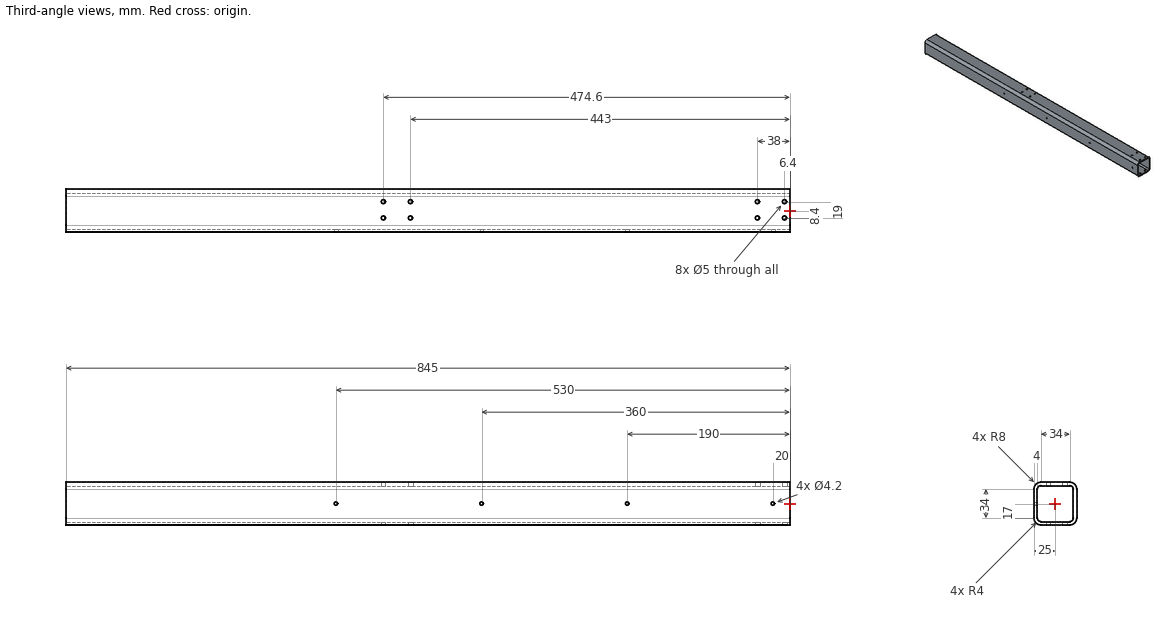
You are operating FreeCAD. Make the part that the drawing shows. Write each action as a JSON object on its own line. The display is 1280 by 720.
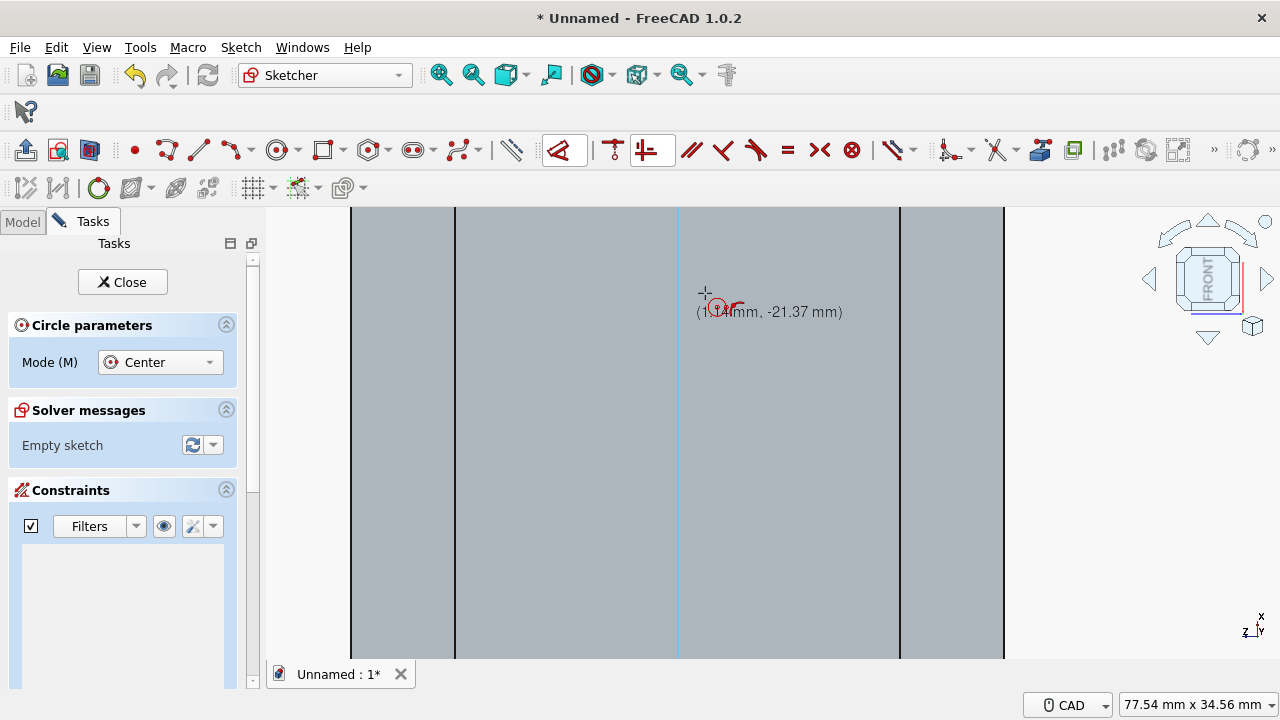
{"action": "scroll", "coordinate": [706, 302], "scroll_direction": "down", "scroll_amount": 16}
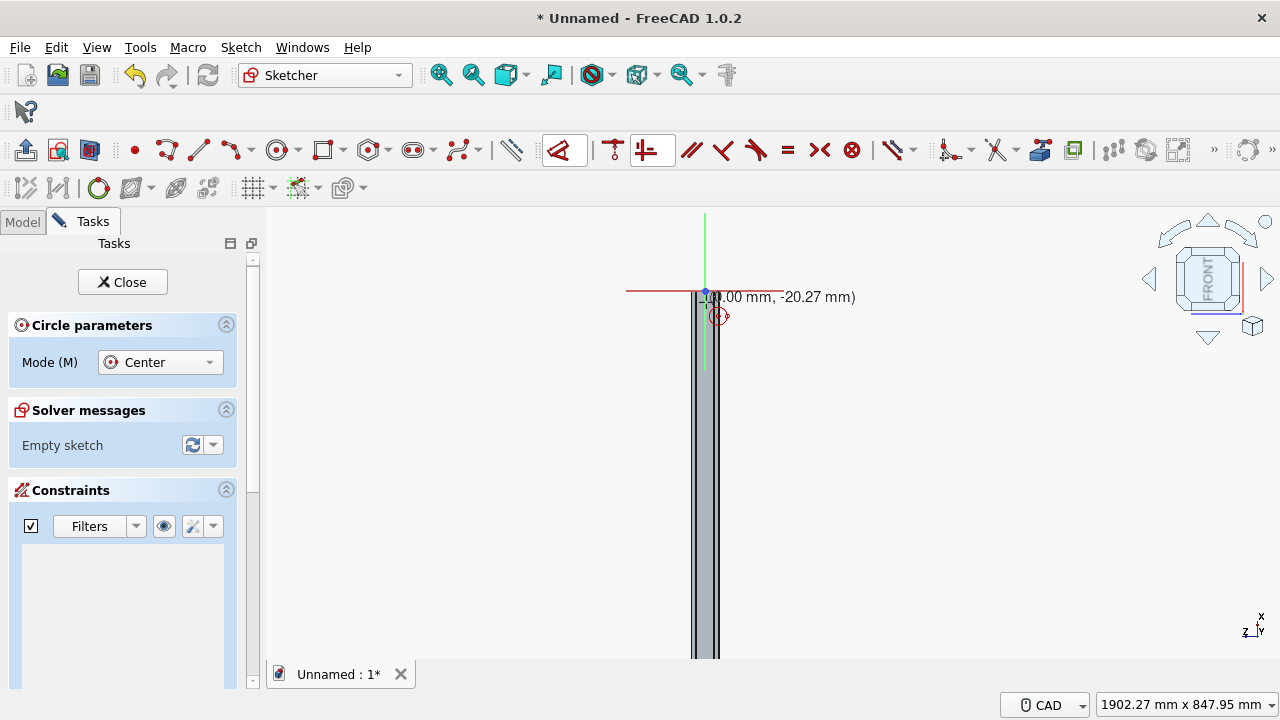
{"action": "scroll", "coordinate": [705, 302], "scroll_direction": "up", "scroll_amount": 2}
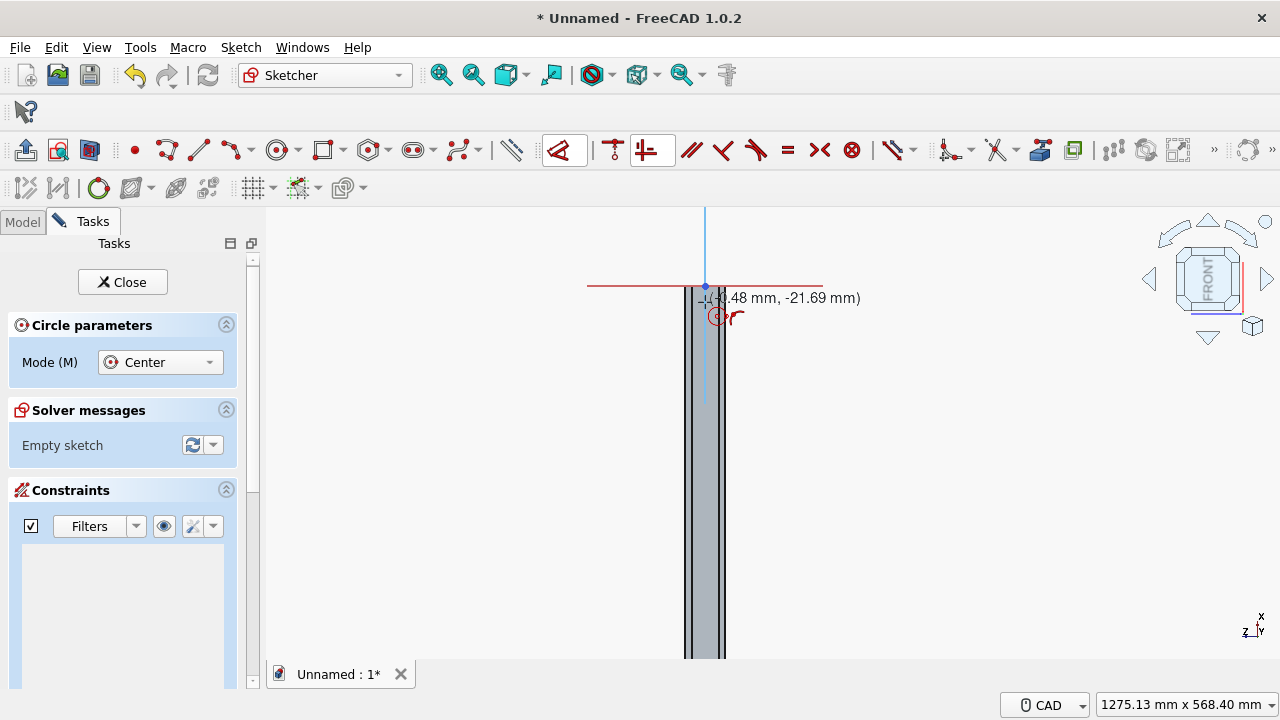
{"action": "left_click", "coordinate": [705, 302]}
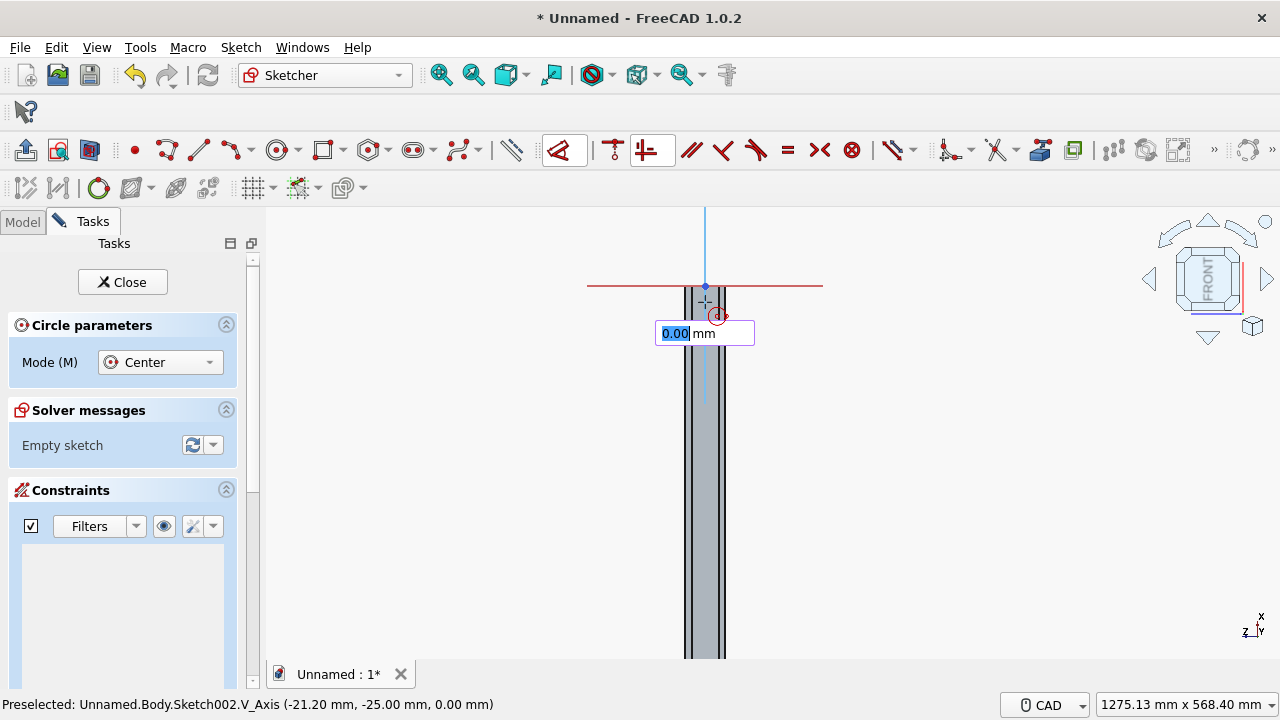
{"action": "scroll", "coordinate": [707, 301], "scroll_direction": "up", "scroll_amount": 12}
{"action": "mouse_move", "coordinate": [700, 304]}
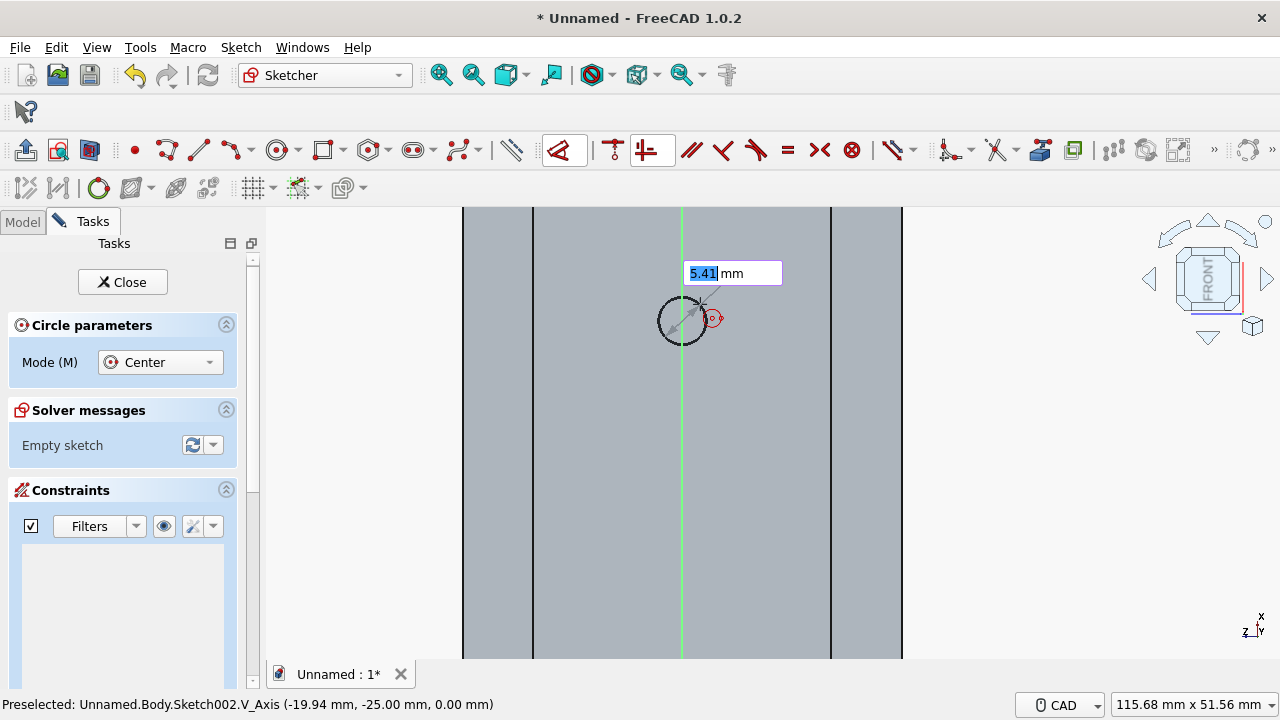
{"action": "type", "text": "4.2"}
{"action": "key", "text": "Return"}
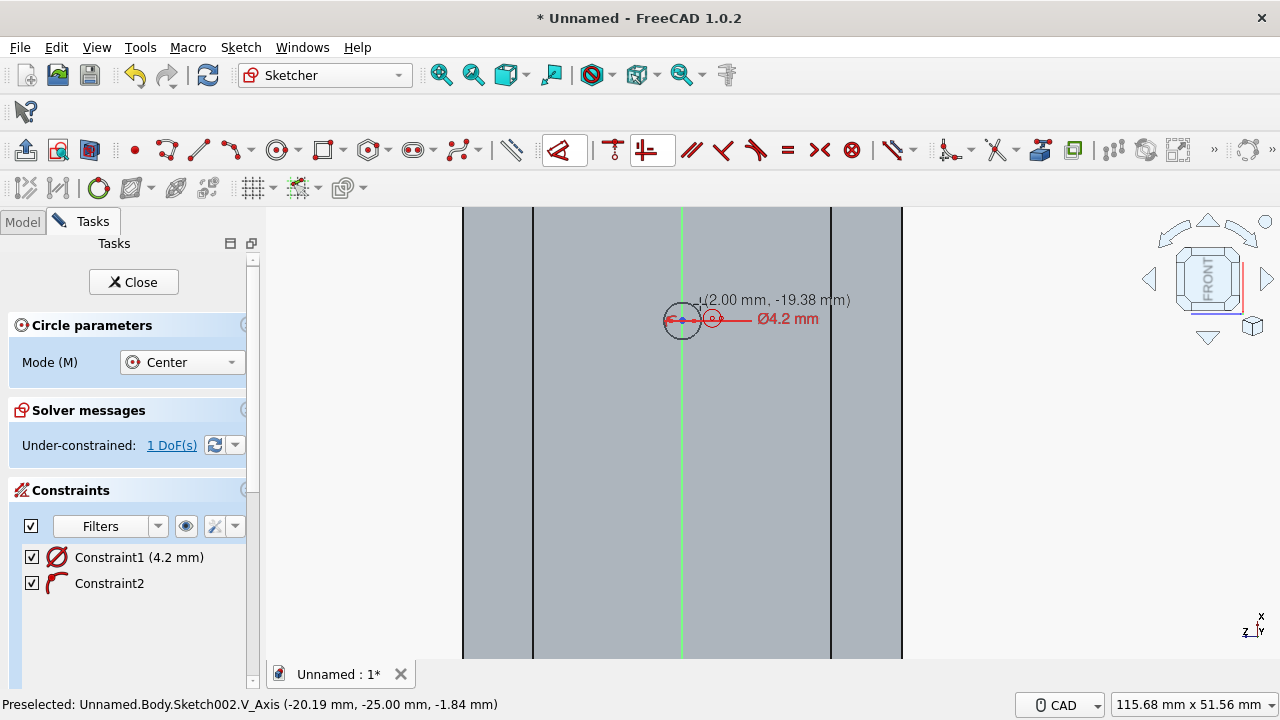
{"action": "scroll", "coordinate": [706, 301], "scroll_direction": "down", "scroll_amount": 14}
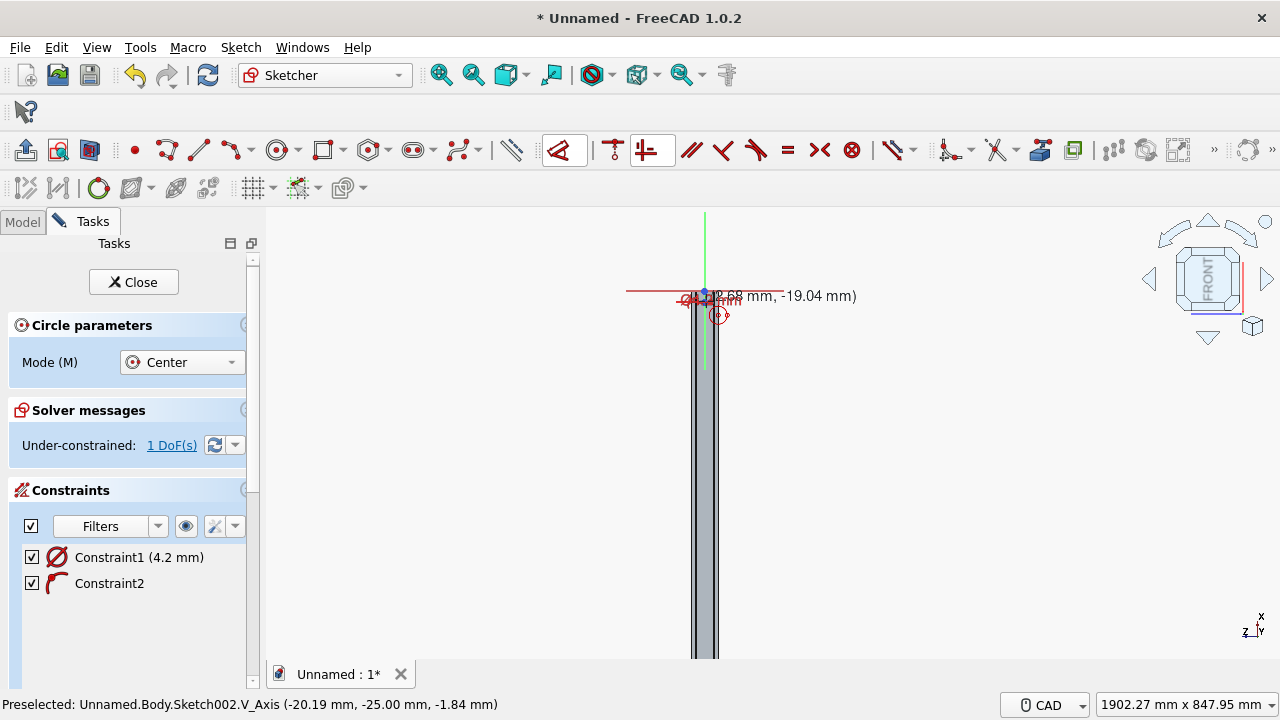
{"action": "scroll", "coordinate": [705, 392], "scroll_direction": "up", "scroll_amount": 16}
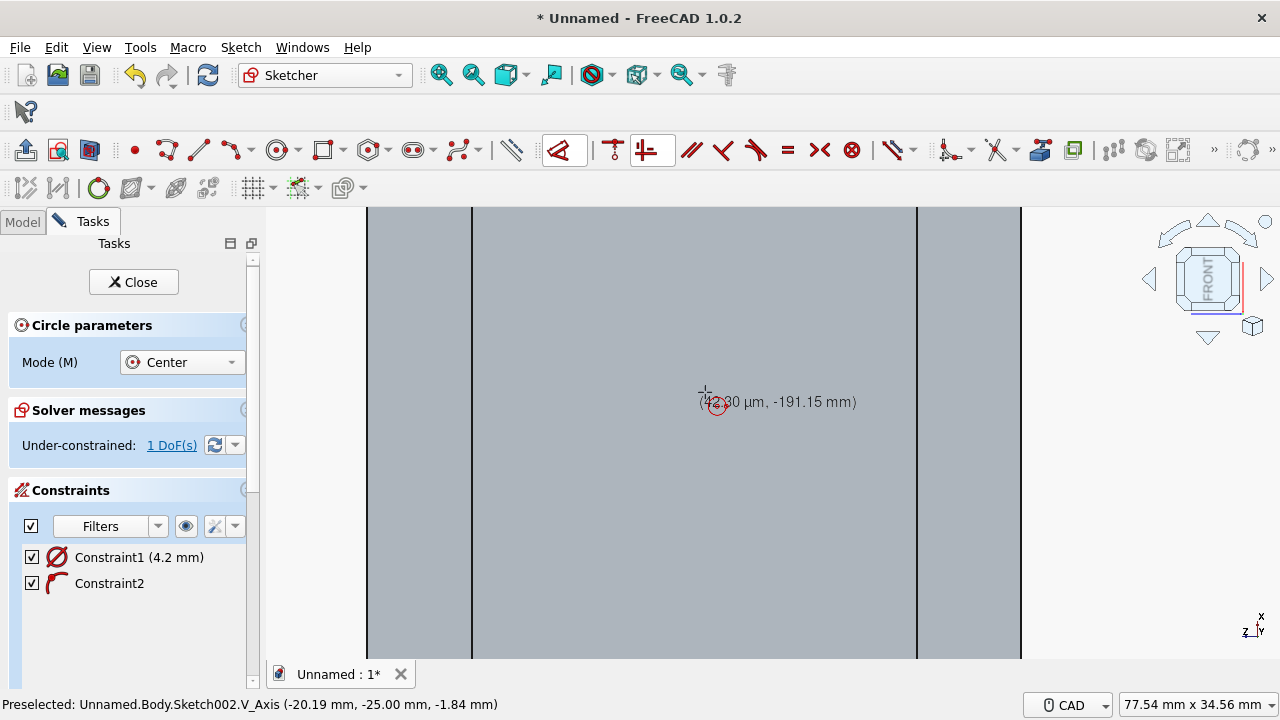
{"action": "scroll", "coordinate": [705, 392], "scroll_direction": "down", "scroll_amount": 16}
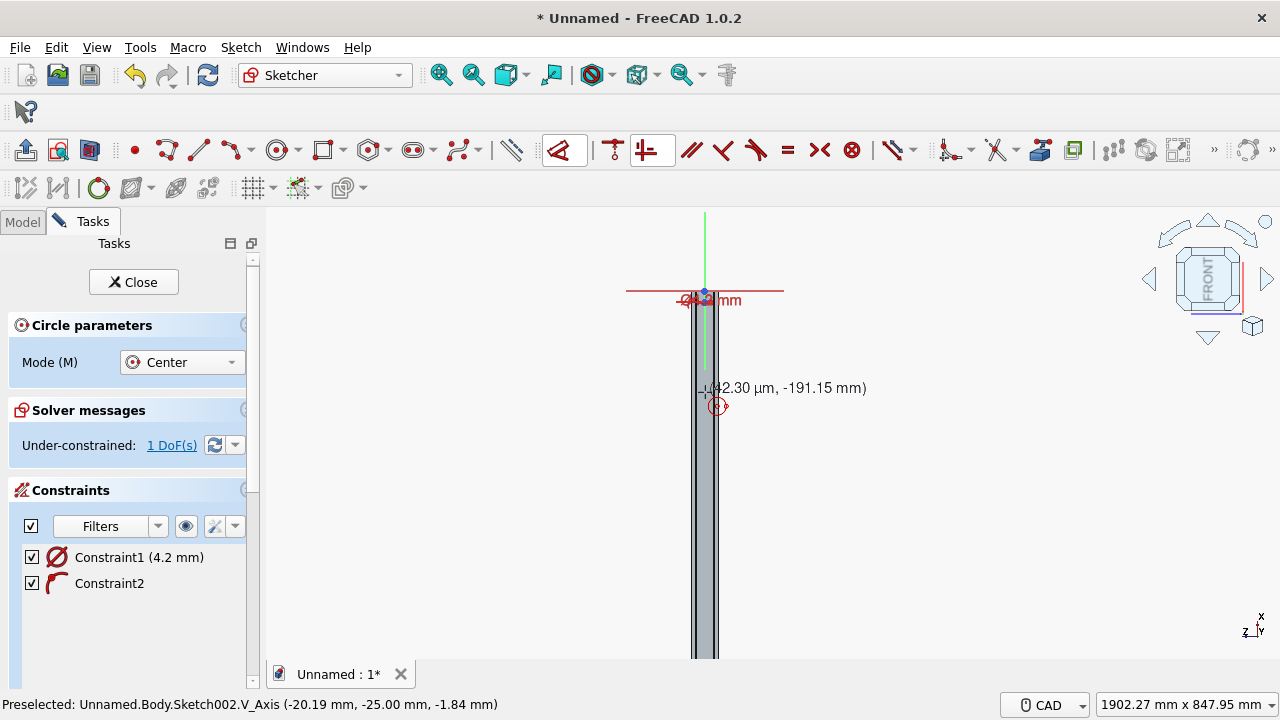
{"action": "left_click", "coordinate": [705, 392]}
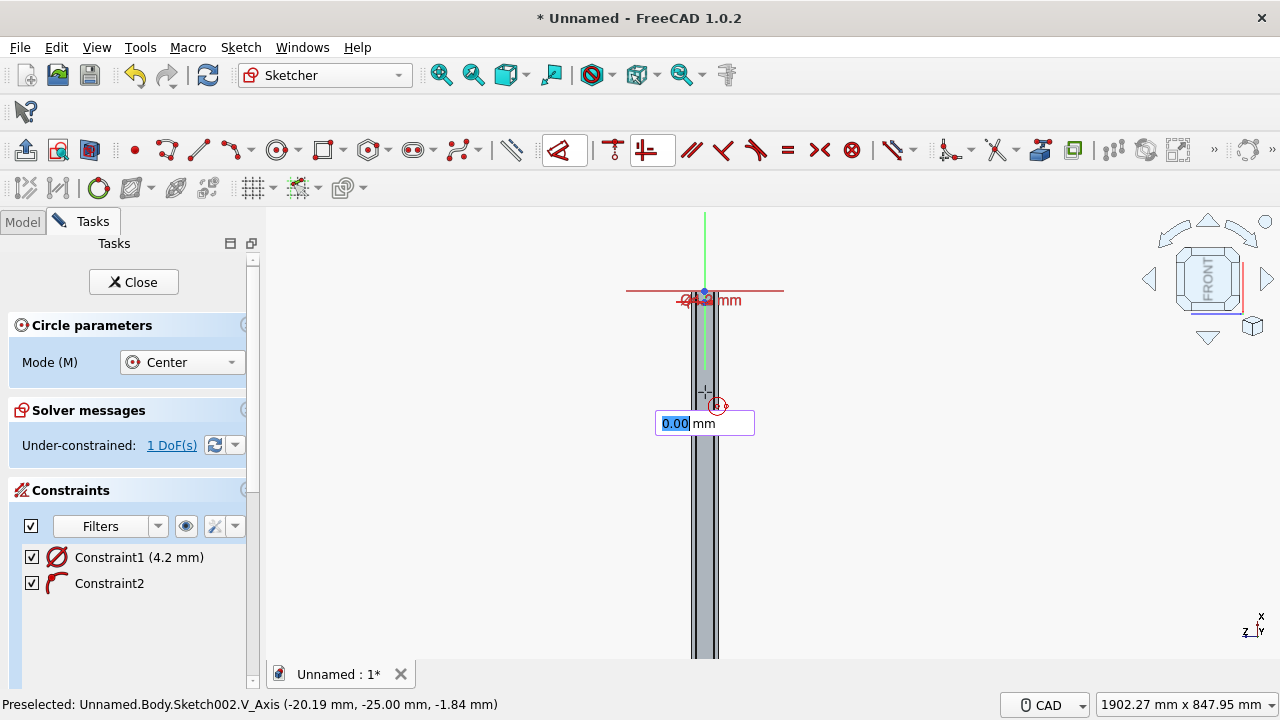
{"action": "scroll", "coordinate": [706, 392], "scroll_direction": "up", "scroll_amount": 14}
{"action": "mouse_move", "coordinate": [700, 386]}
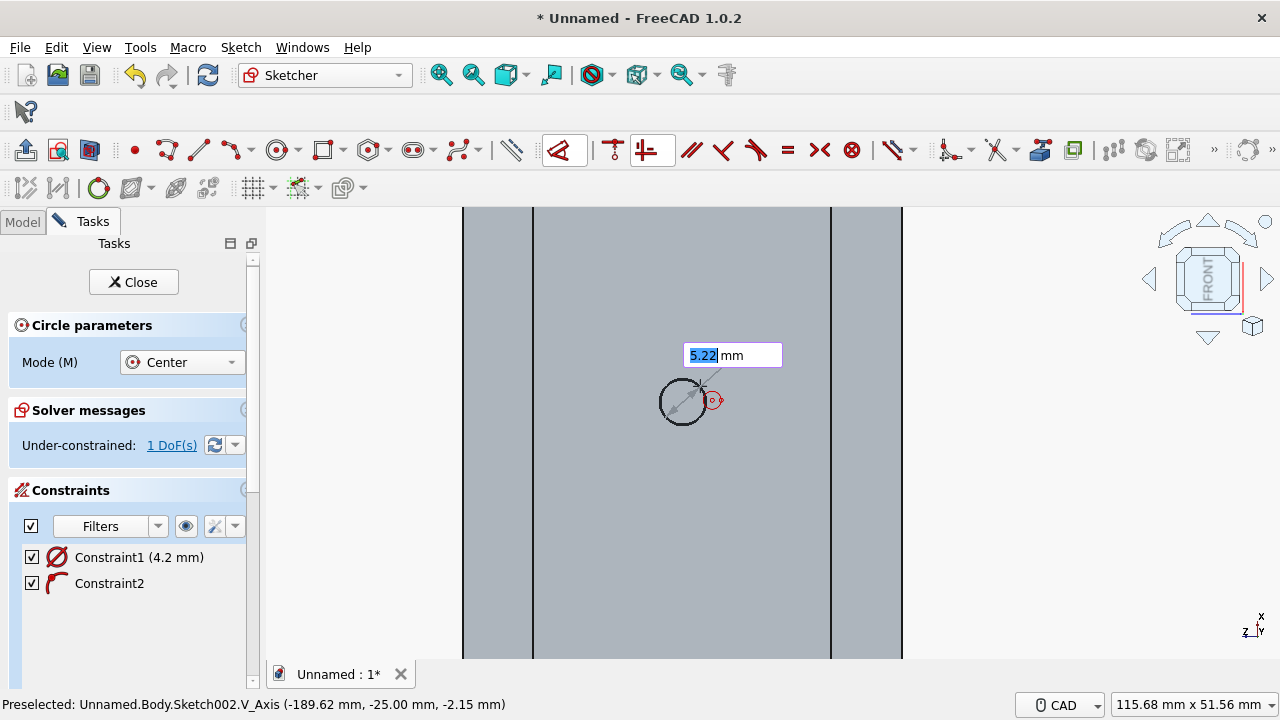
{"action": "type", "text": "4.2"}
{"action": "key", "text": "Return"}